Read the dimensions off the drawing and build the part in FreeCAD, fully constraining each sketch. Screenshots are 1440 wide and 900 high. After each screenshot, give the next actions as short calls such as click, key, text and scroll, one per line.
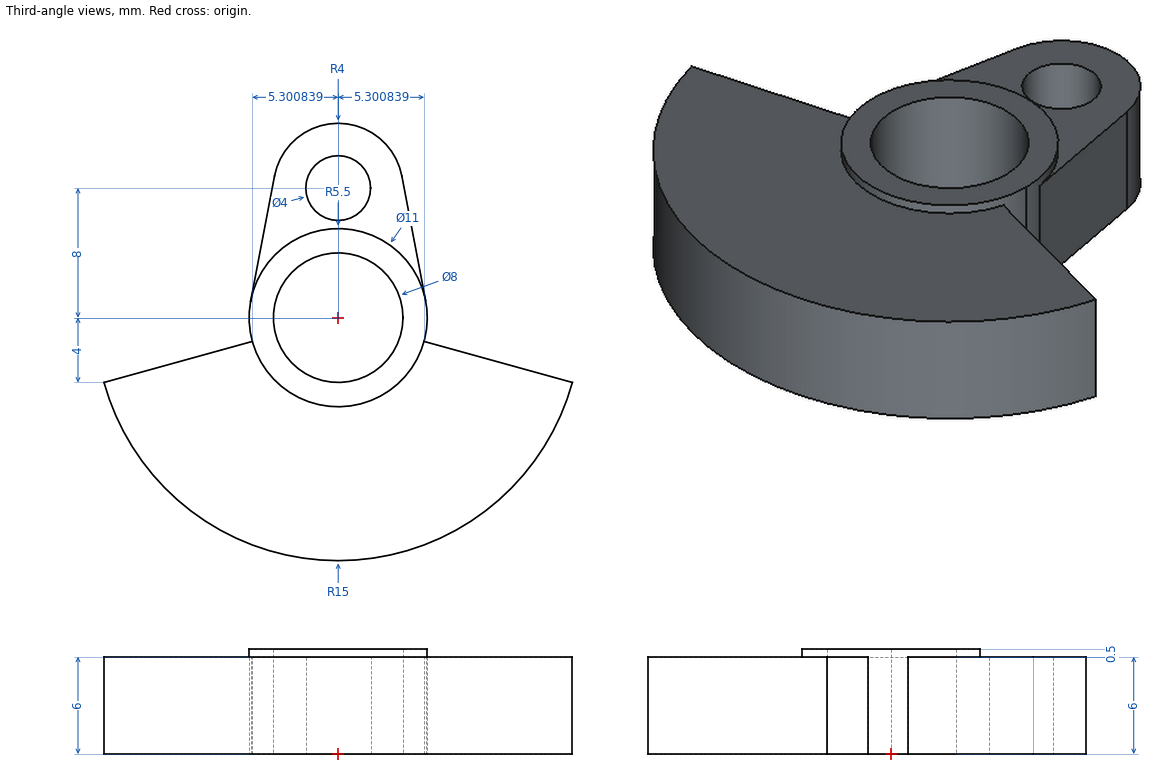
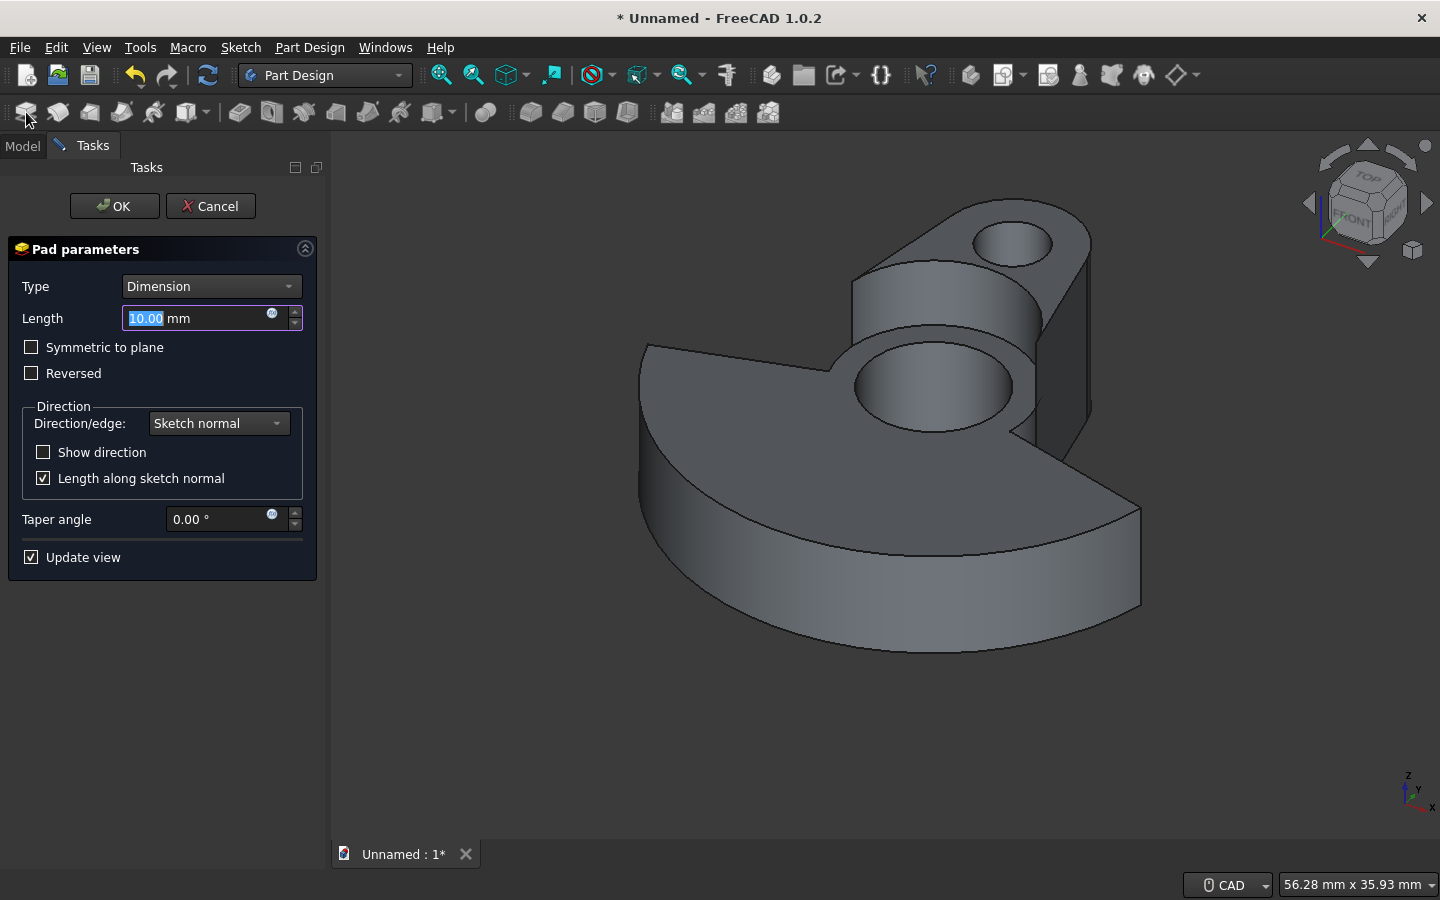
text(6)
key(Tab)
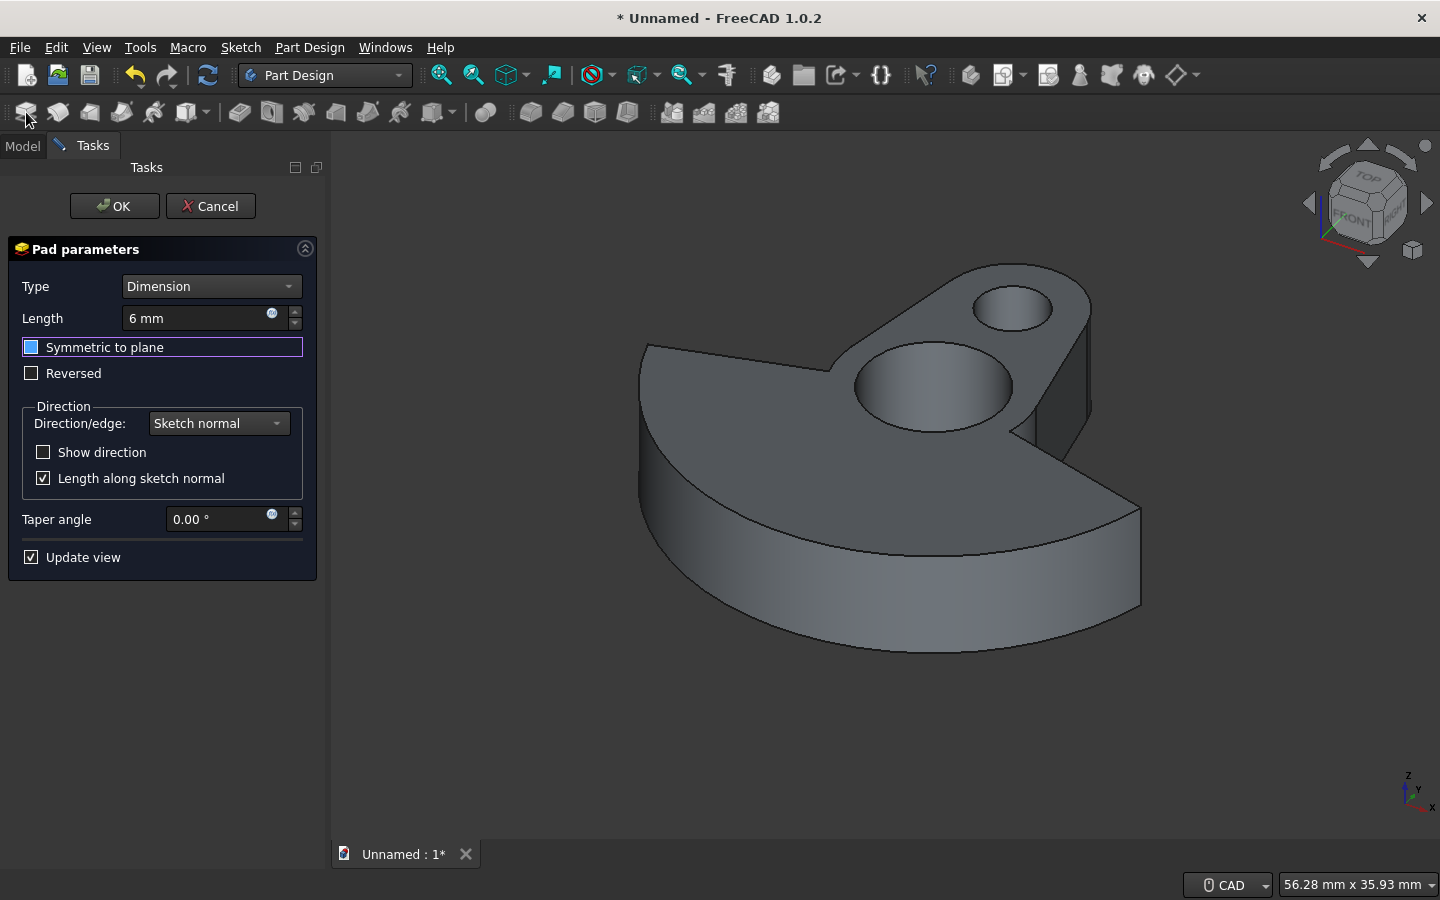
click(115, 206)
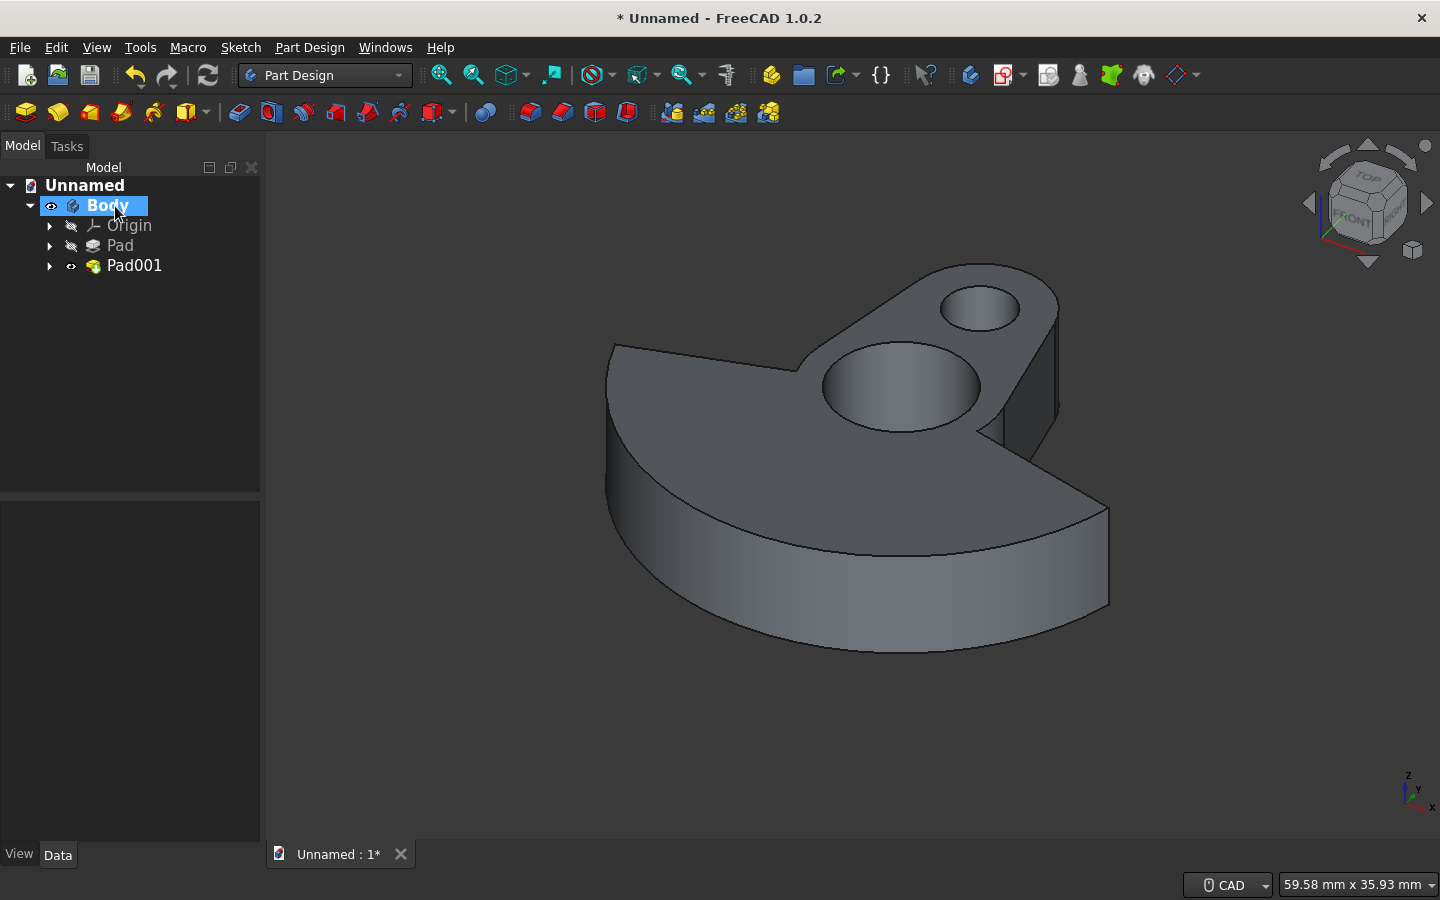
click(811, 476)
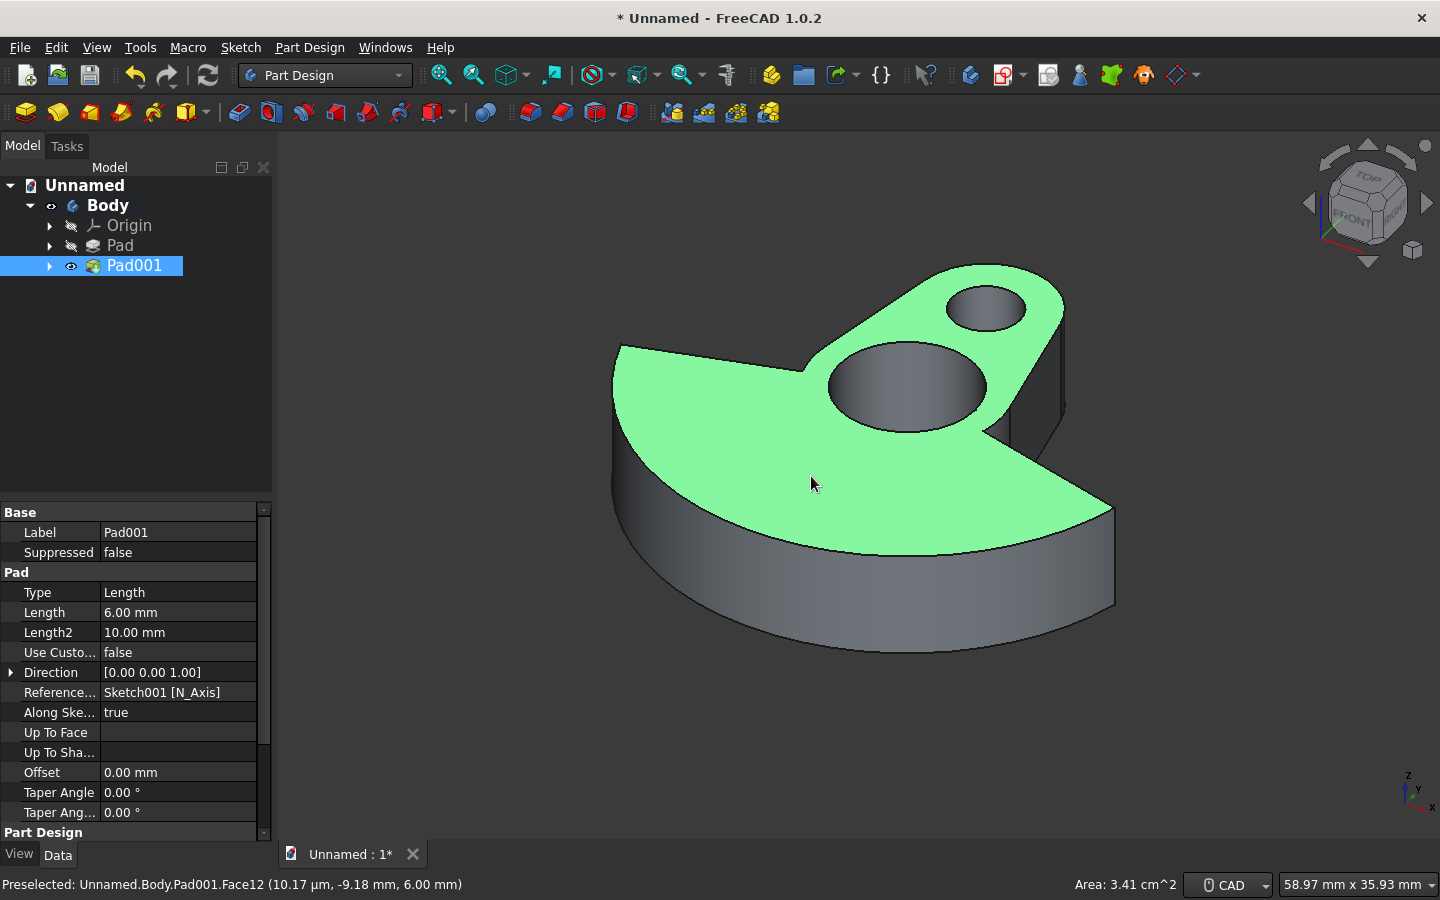
click(1004, 76)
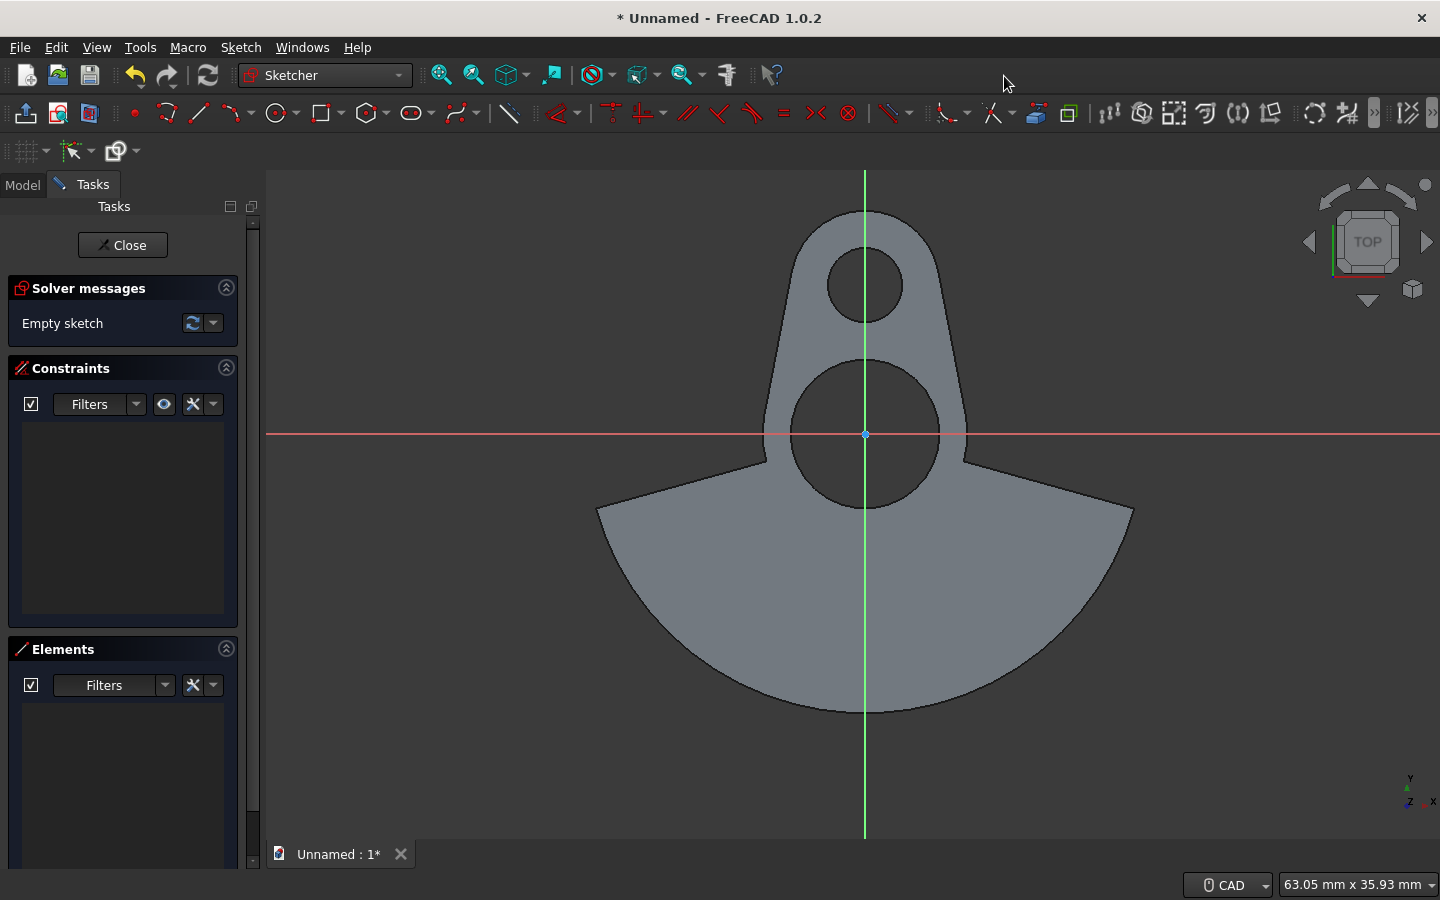
scroll(931, 377, up, 4)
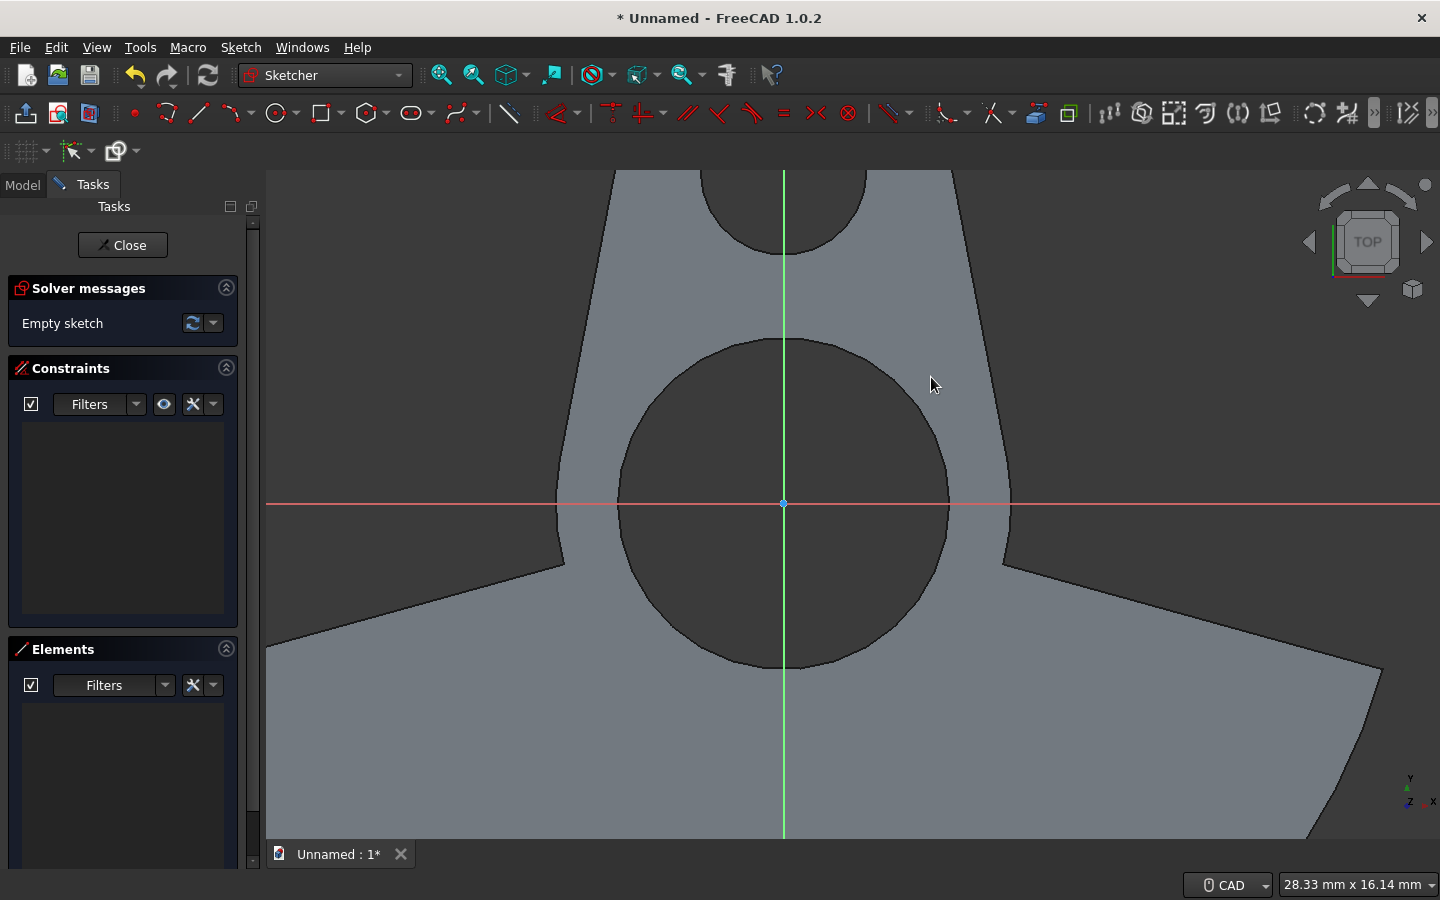
click(276, 114)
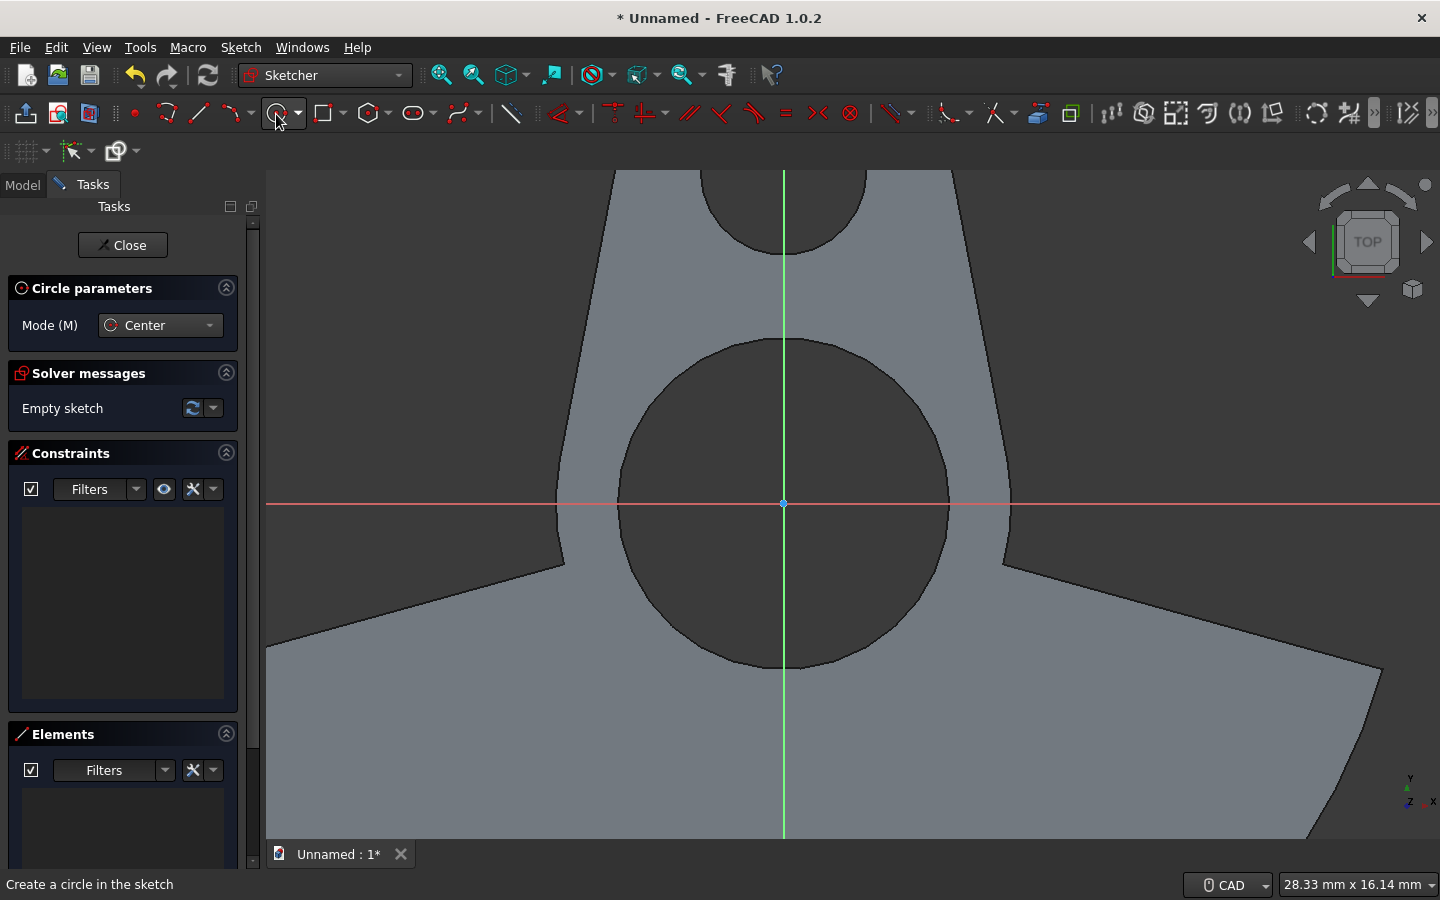
click(784, 504)
click(945, 342)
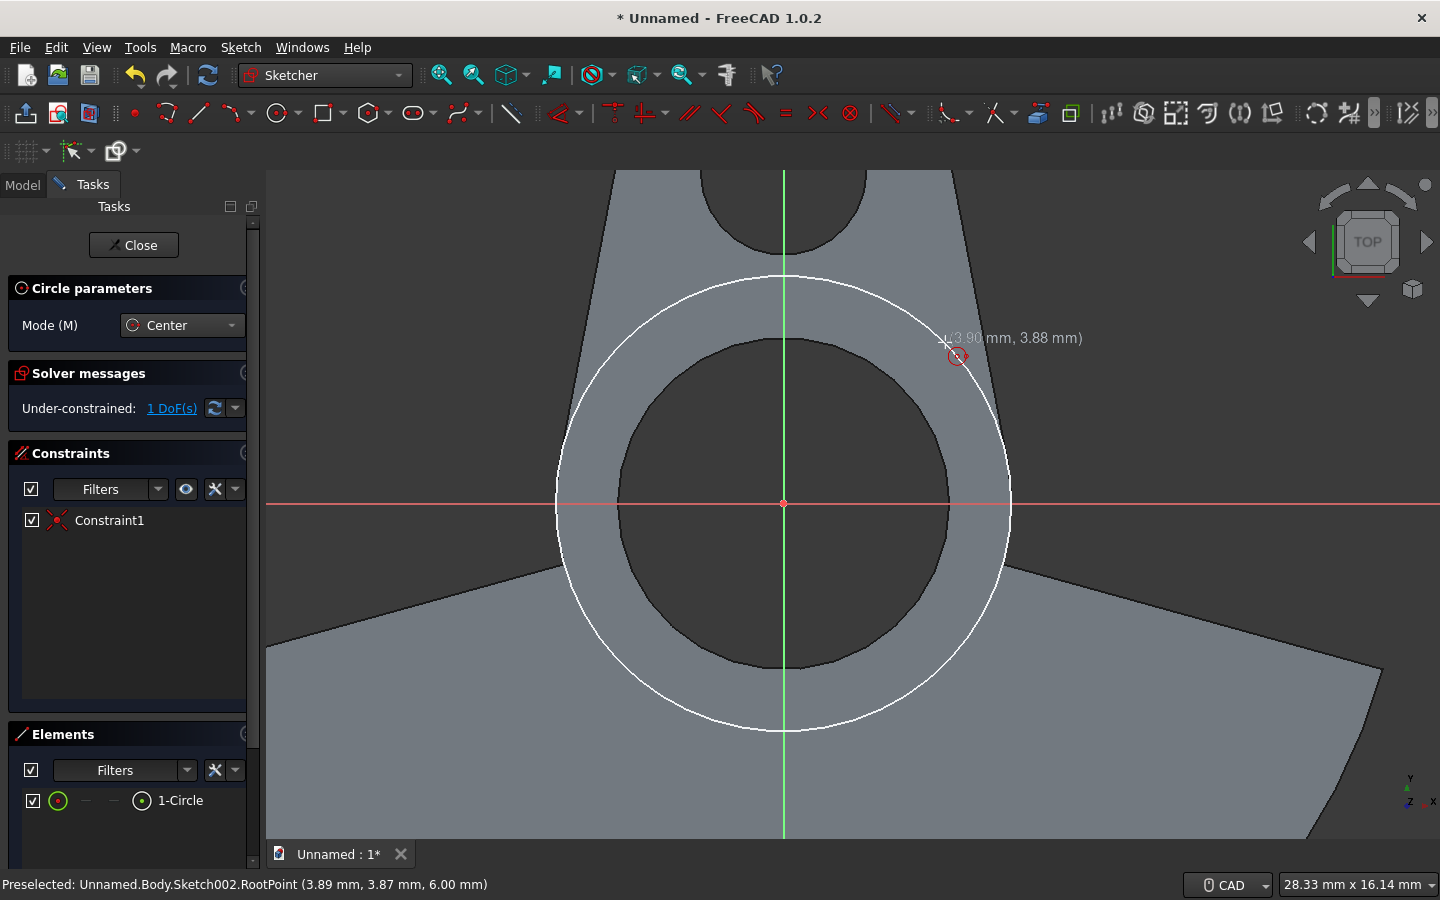
click(784, 504)
click(901, 386)
key(Escape)